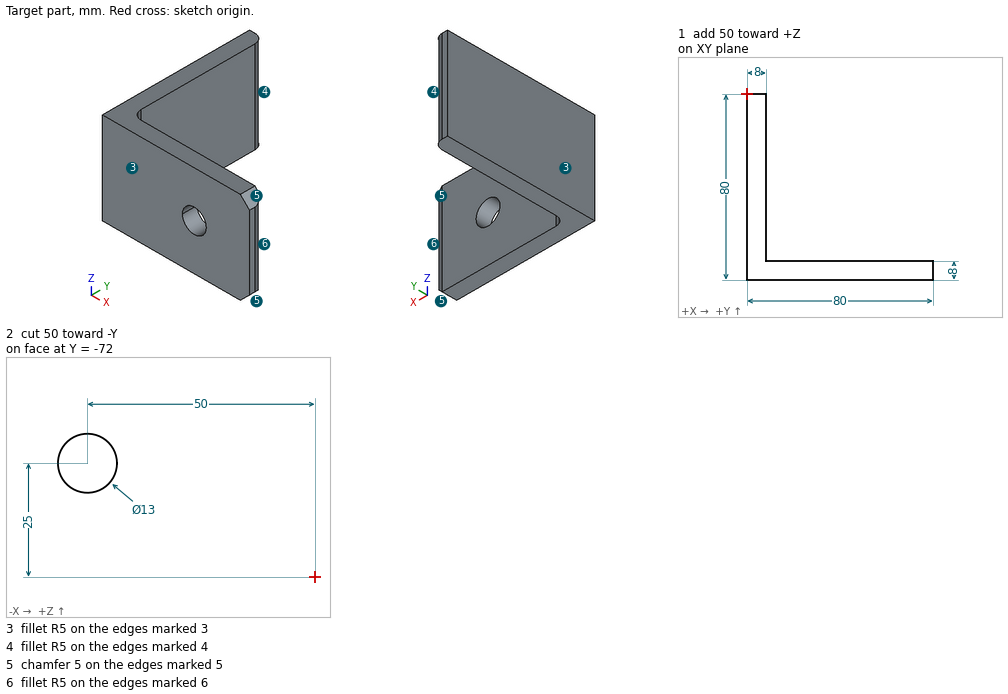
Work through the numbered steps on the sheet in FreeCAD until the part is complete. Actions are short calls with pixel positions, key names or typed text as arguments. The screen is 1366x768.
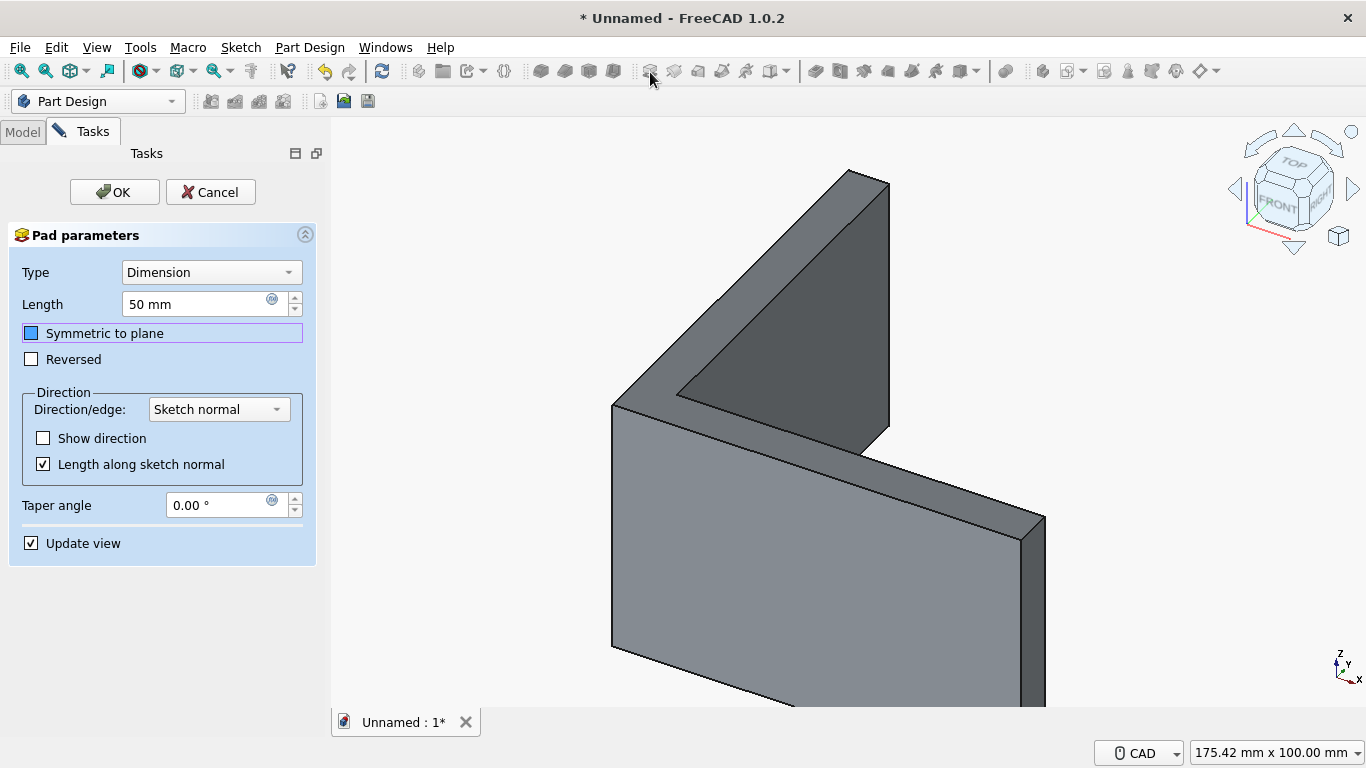
click(115, 192)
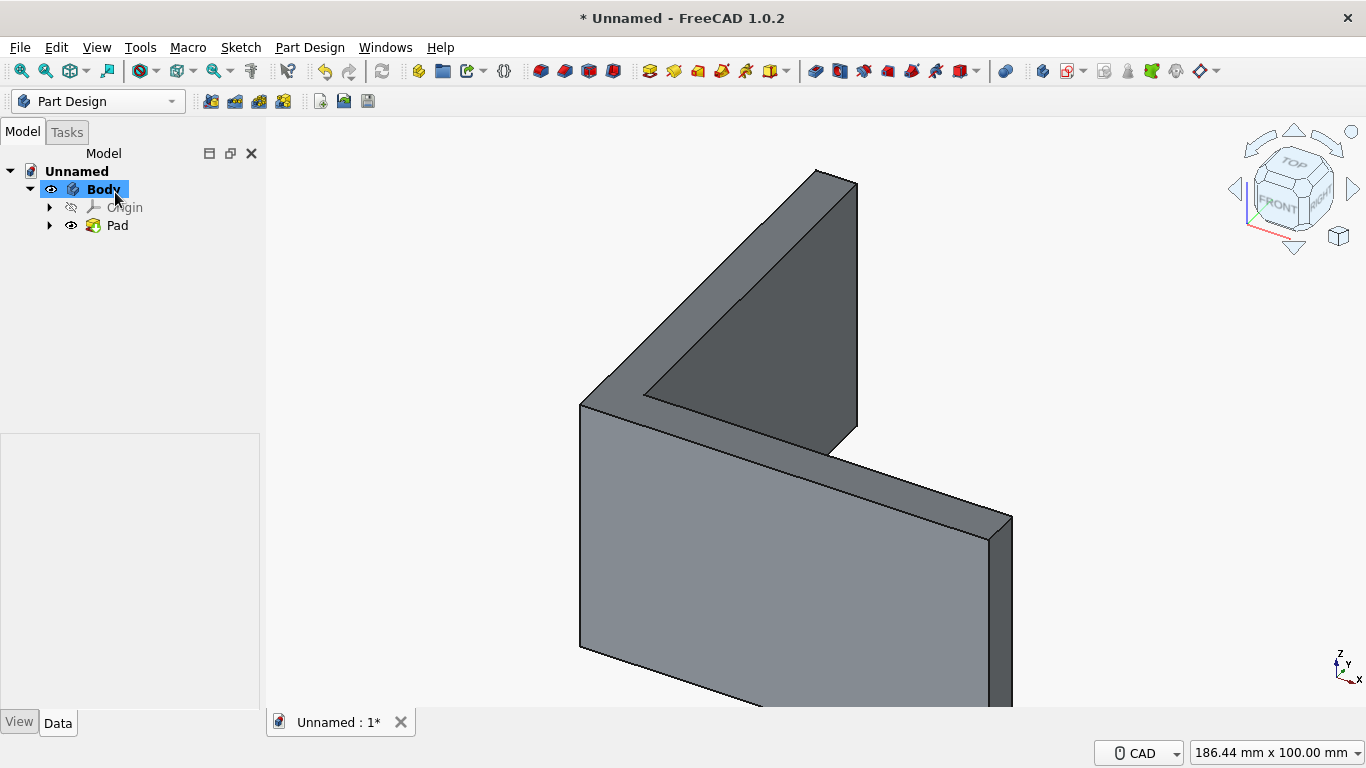
click(22, 72)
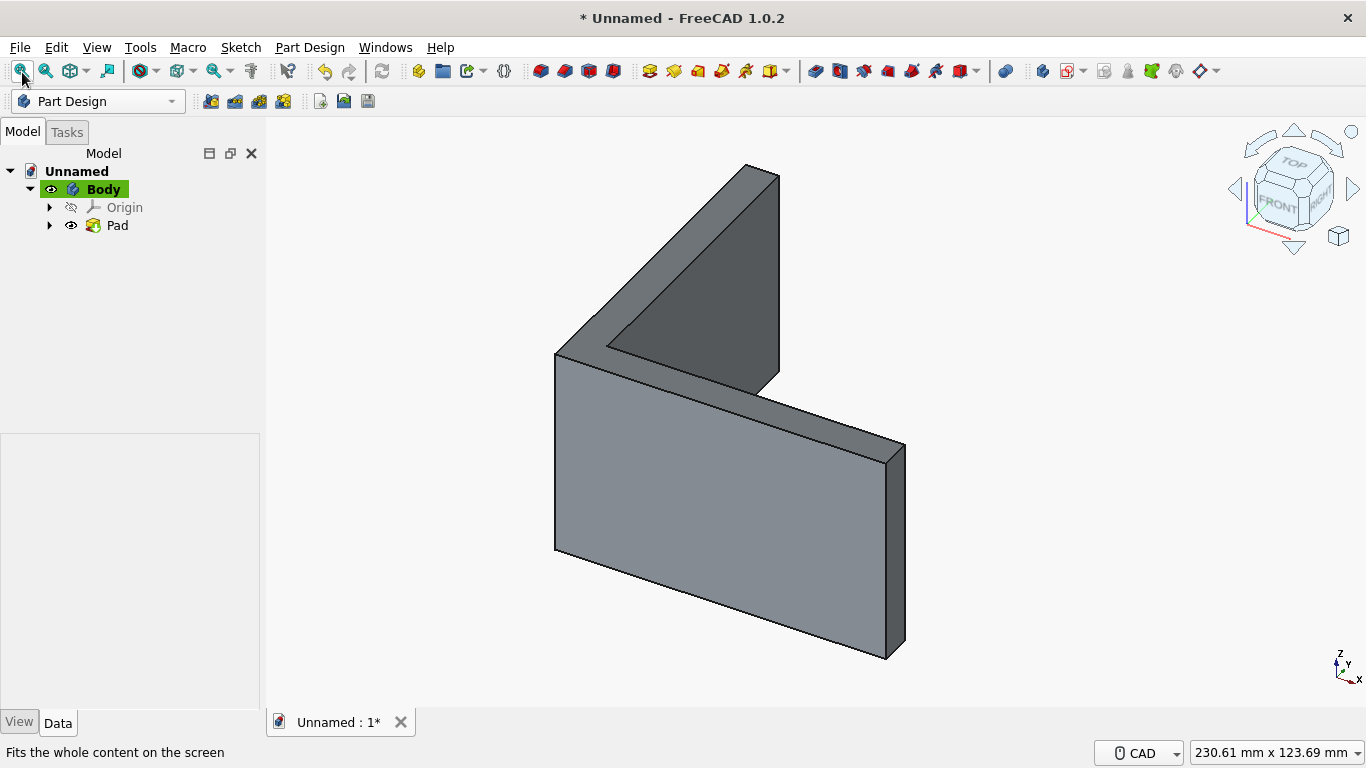
key(4)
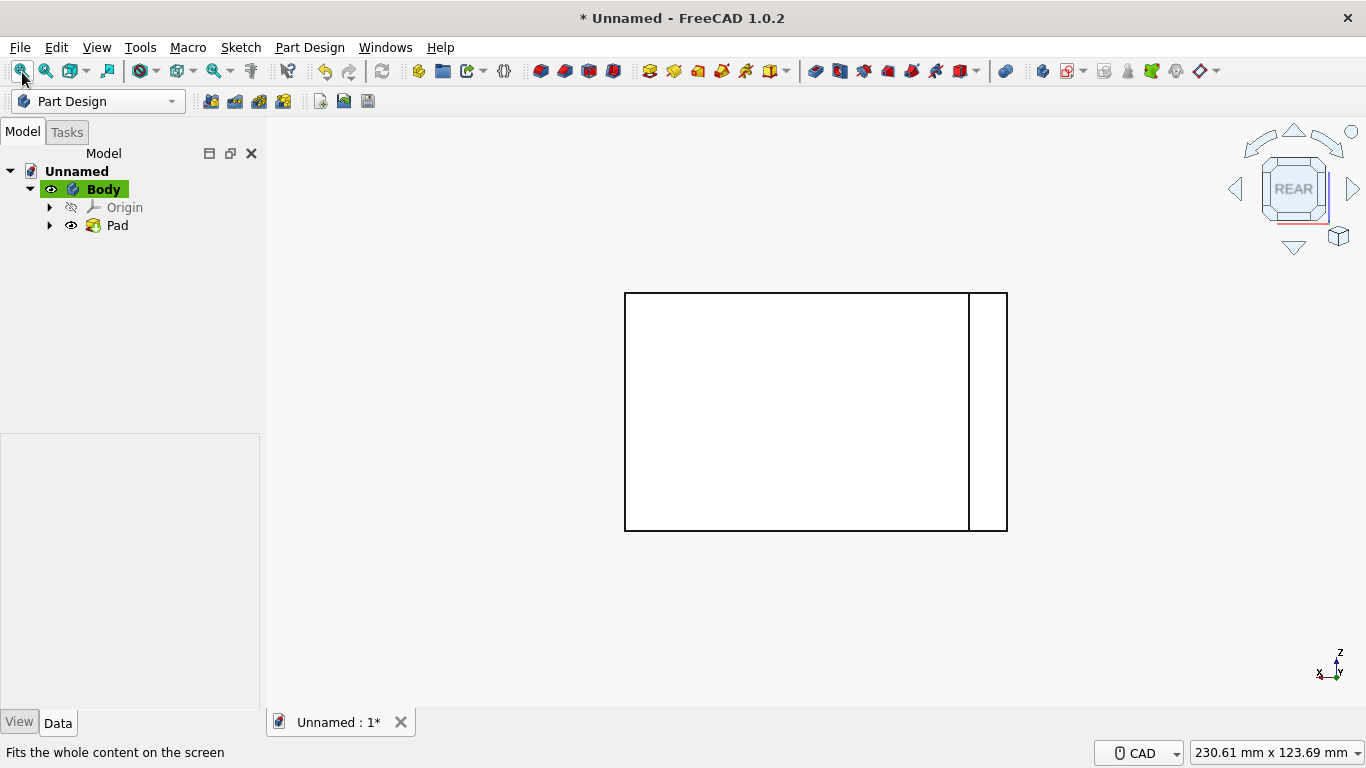
click(22, 72)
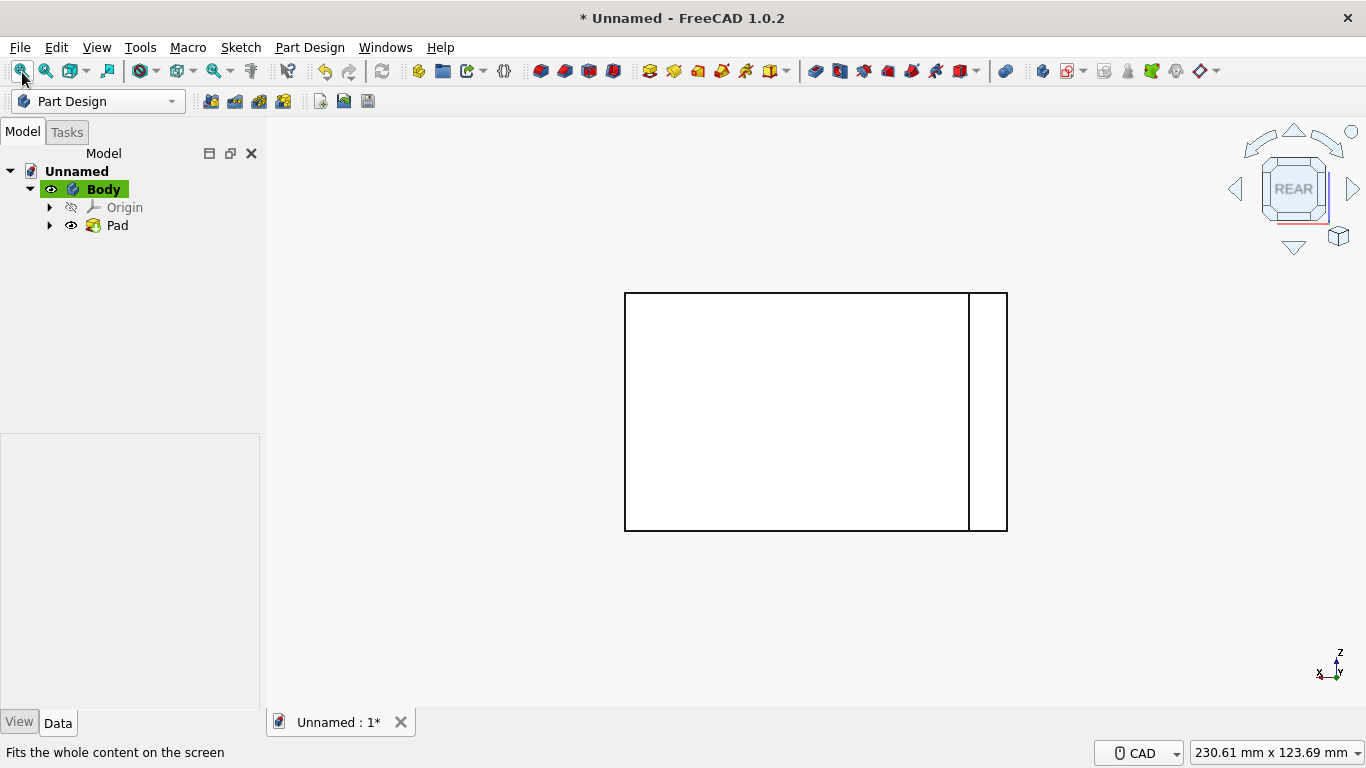
click(748, 411)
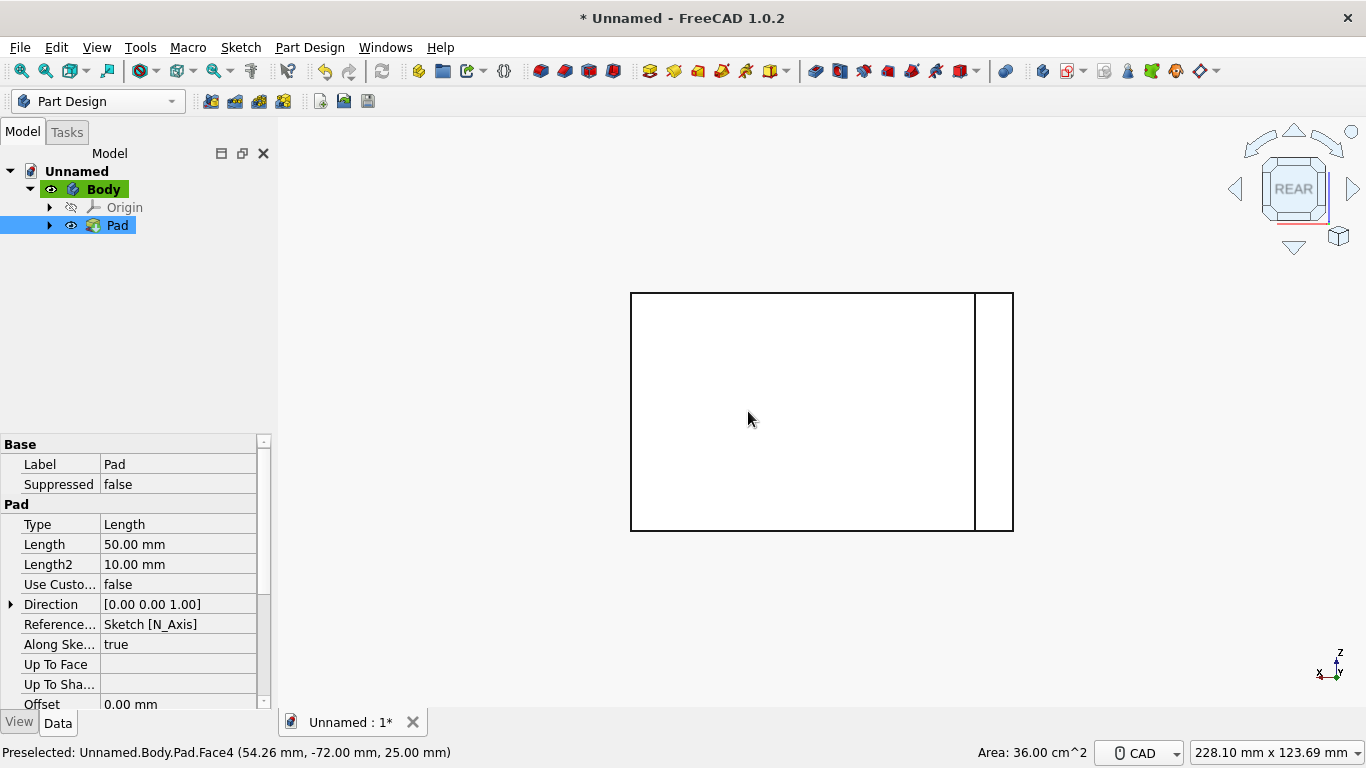
click(1068, 72)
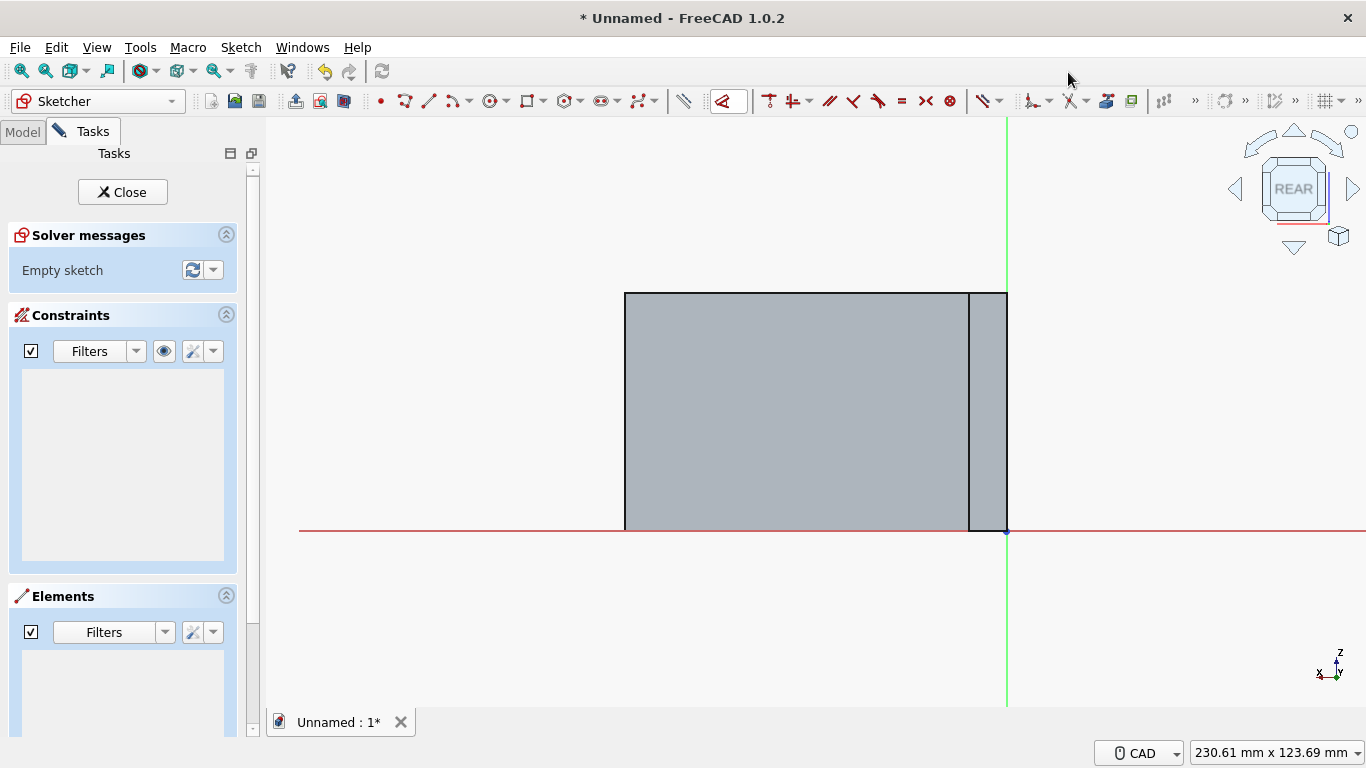
scroll(772, 412, up, 9)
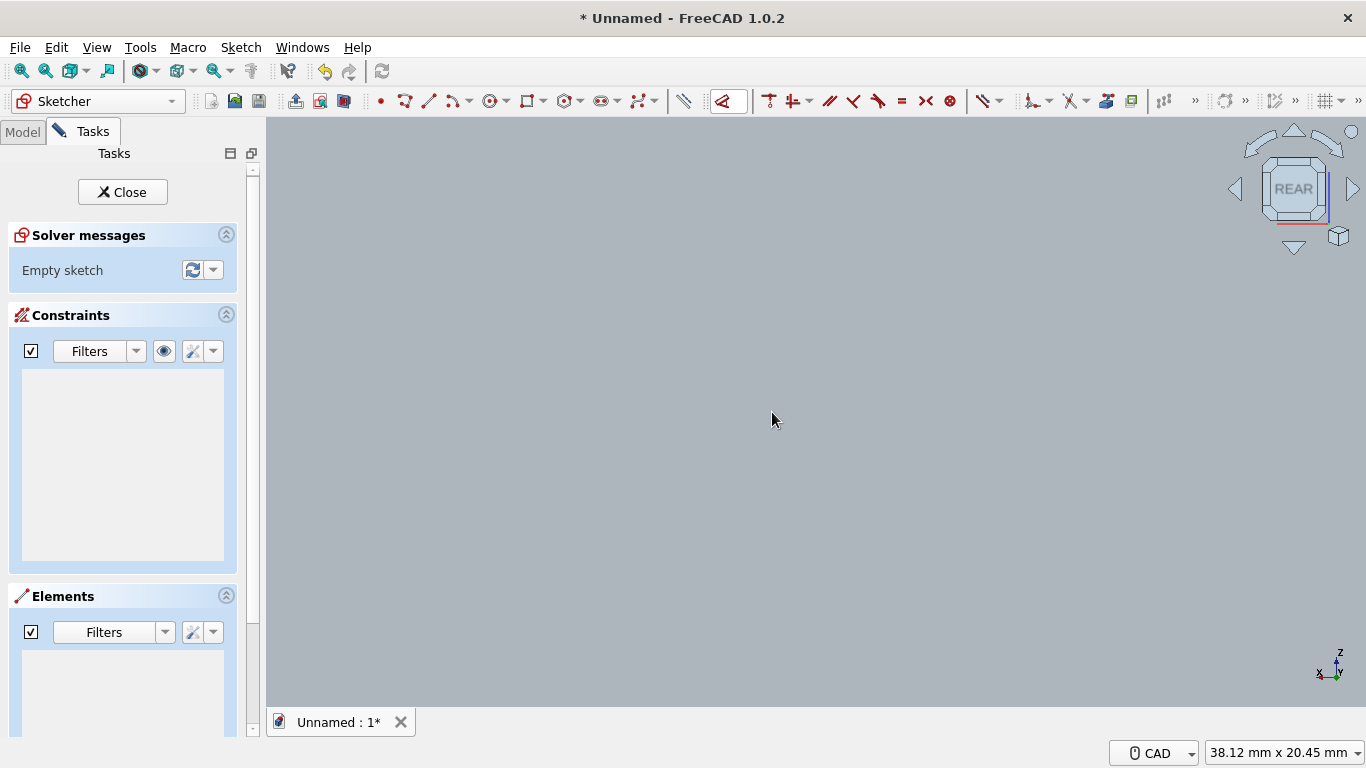
key(g)
key(c)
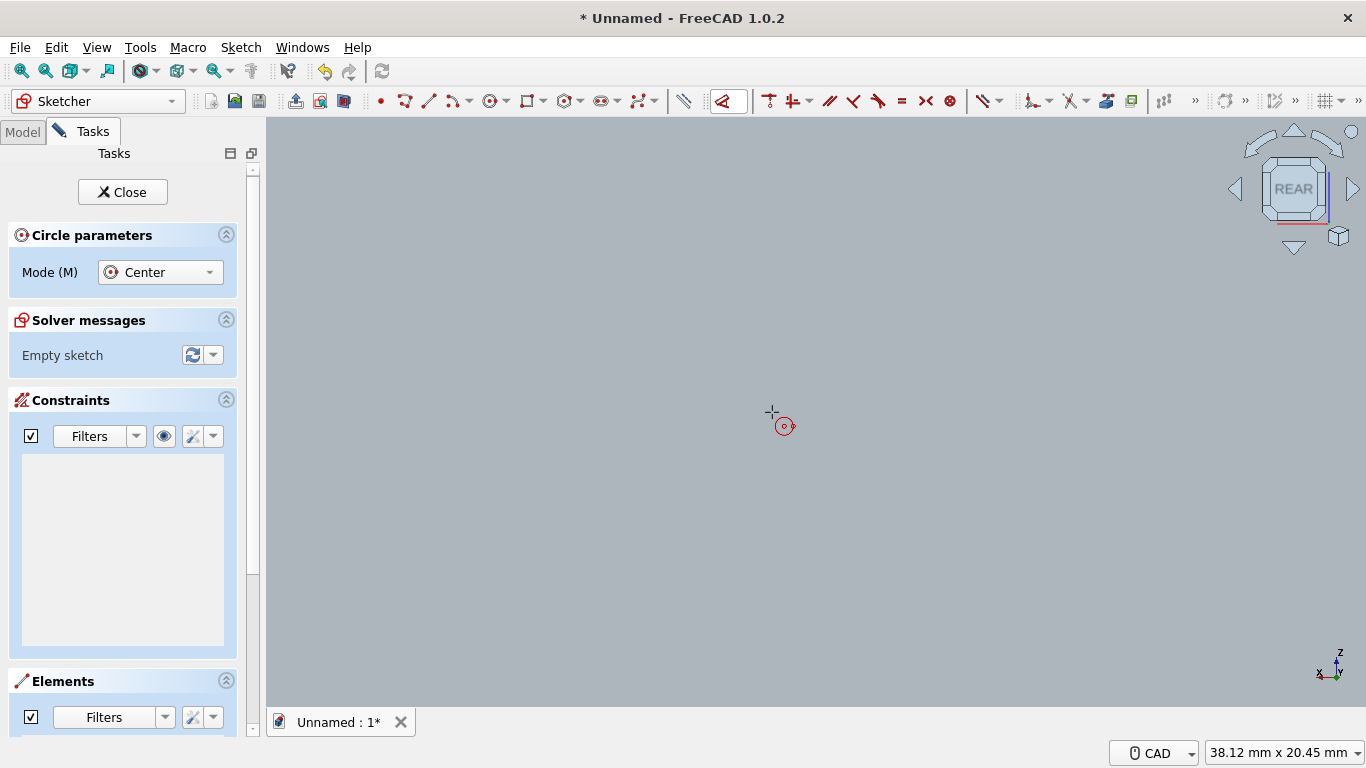
click(747, 409)
click(880, 277)
key(Escape)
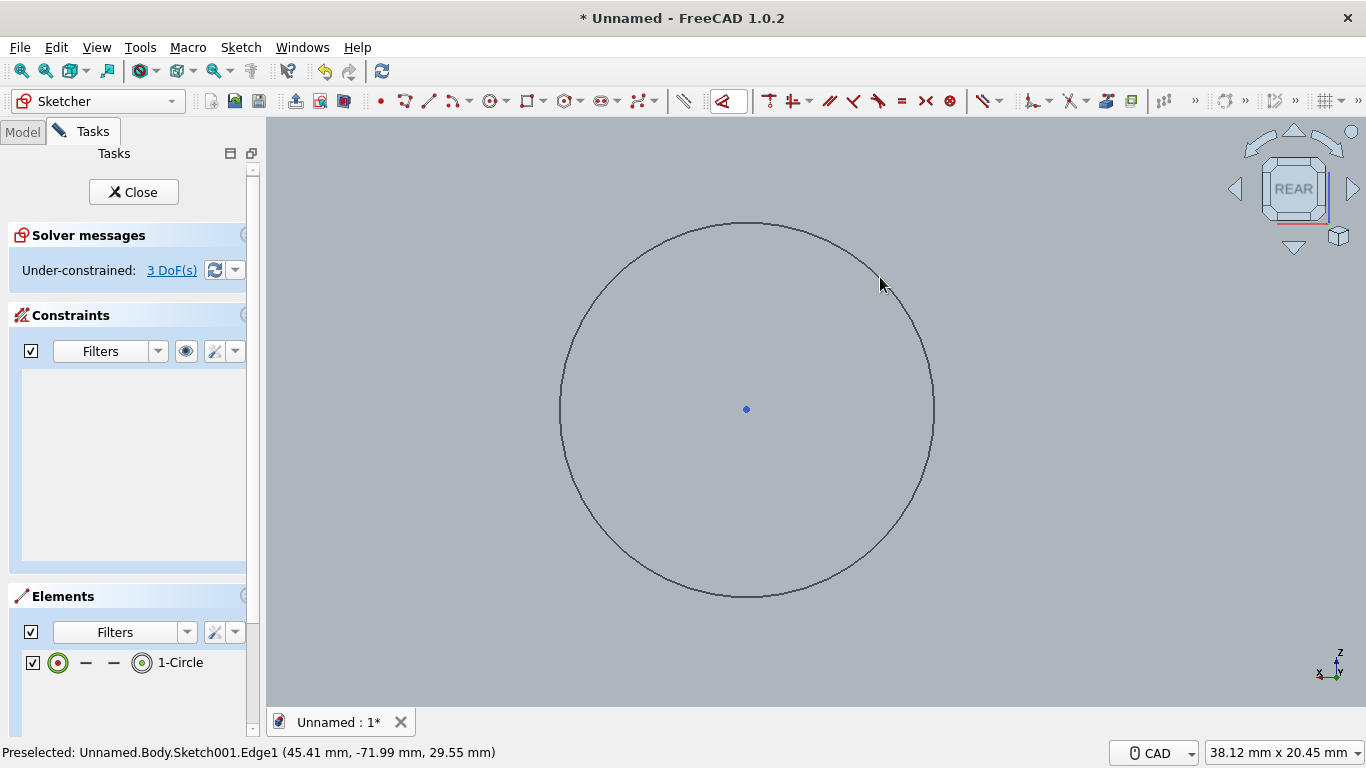
click(879, 277)